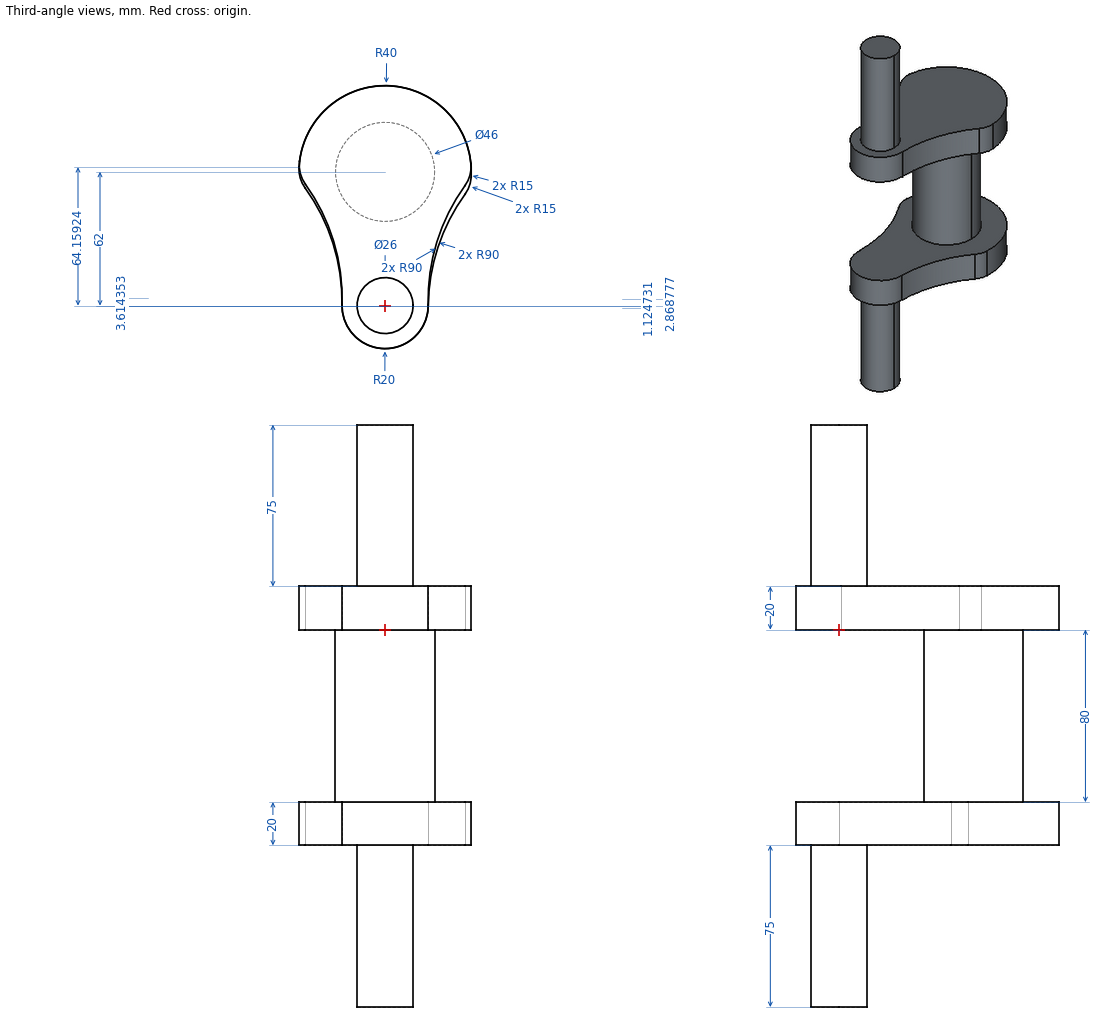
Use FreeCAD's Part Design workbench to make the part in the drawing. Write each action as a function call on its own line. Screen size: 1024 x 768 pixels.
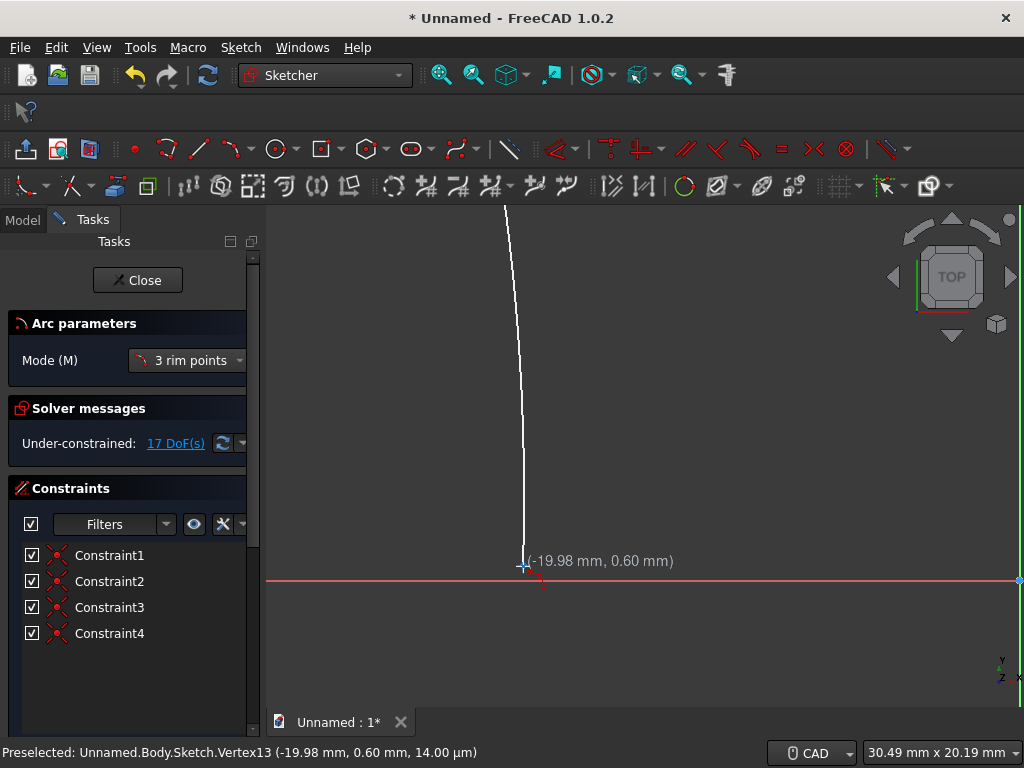
scroll(521, 567, down, 11)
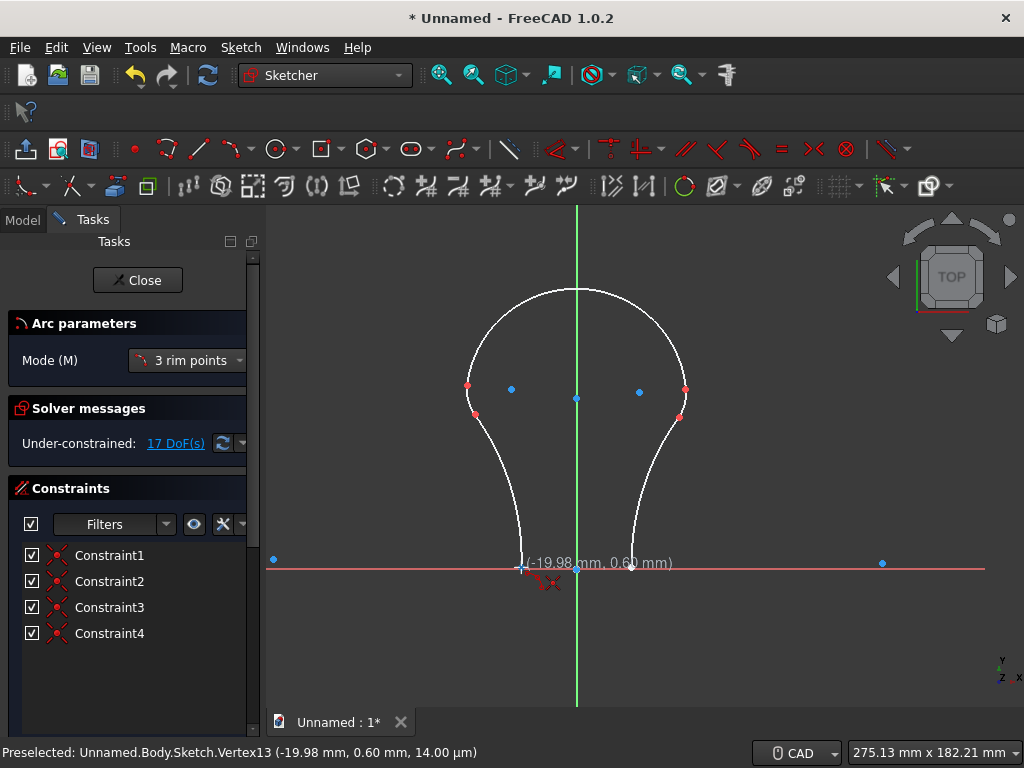
scroll(632, 568, up, 13)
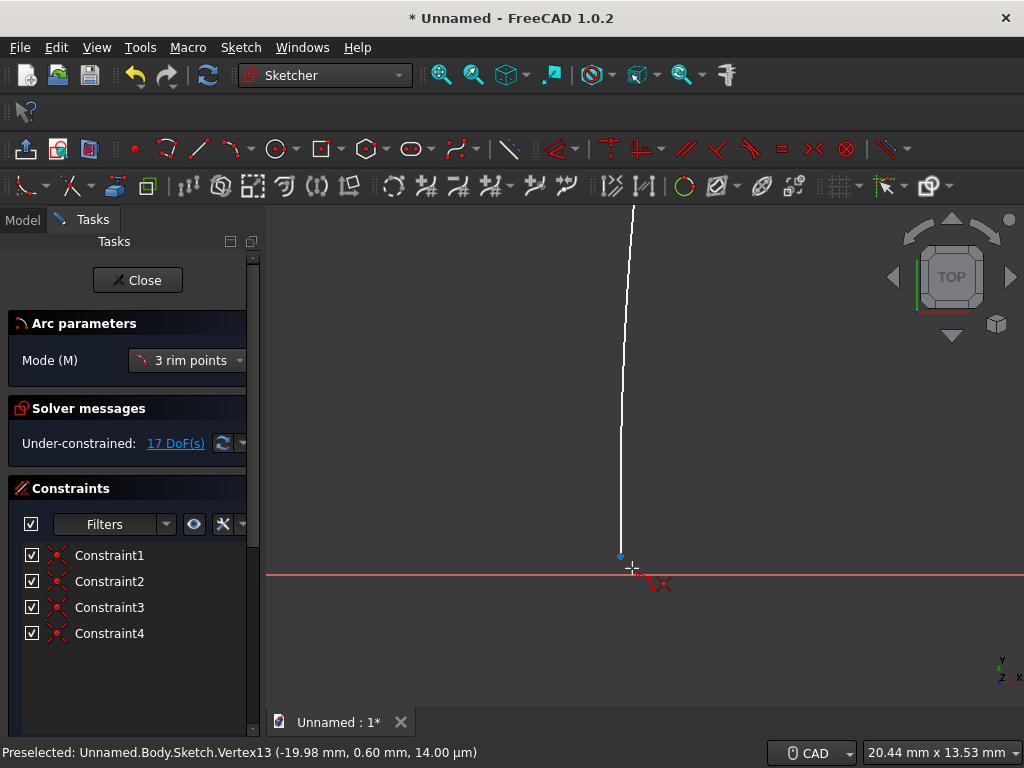
click(621, 557)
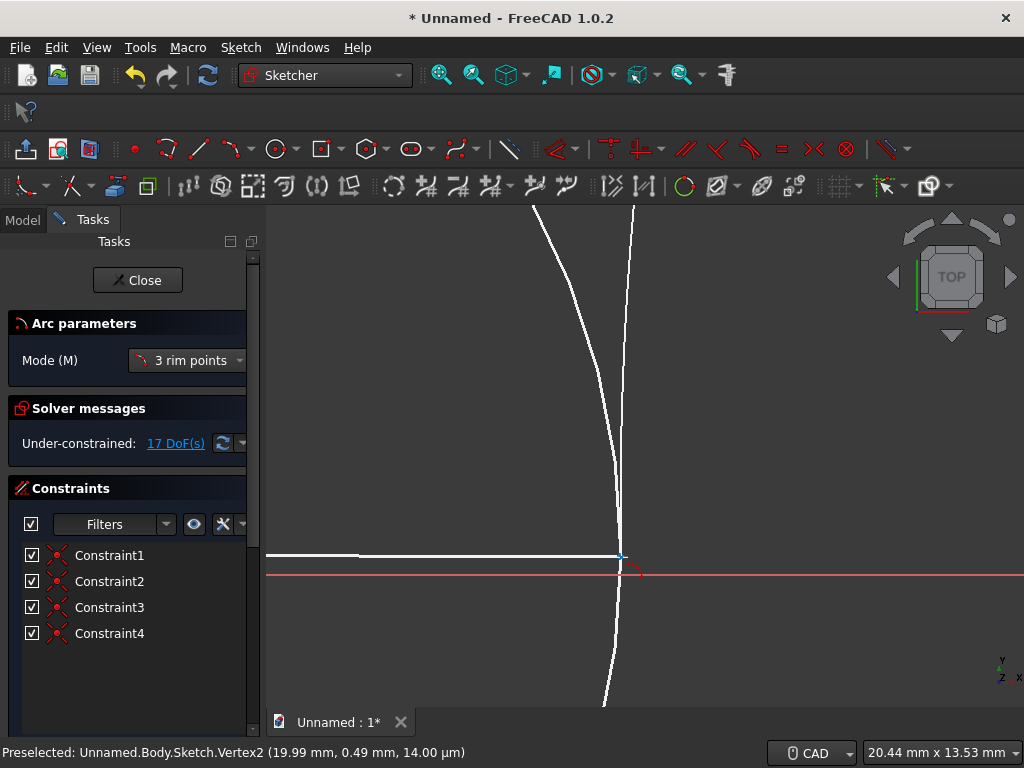
scroll(632, 568, down, 13)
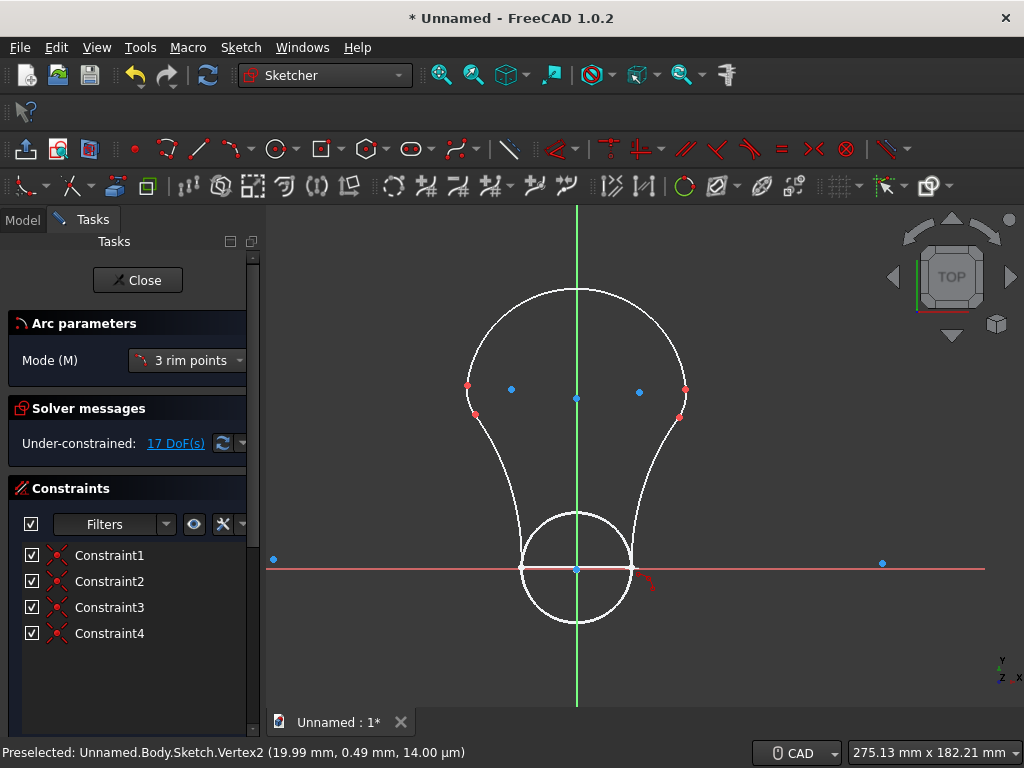
click(559, 621)
key(Escape)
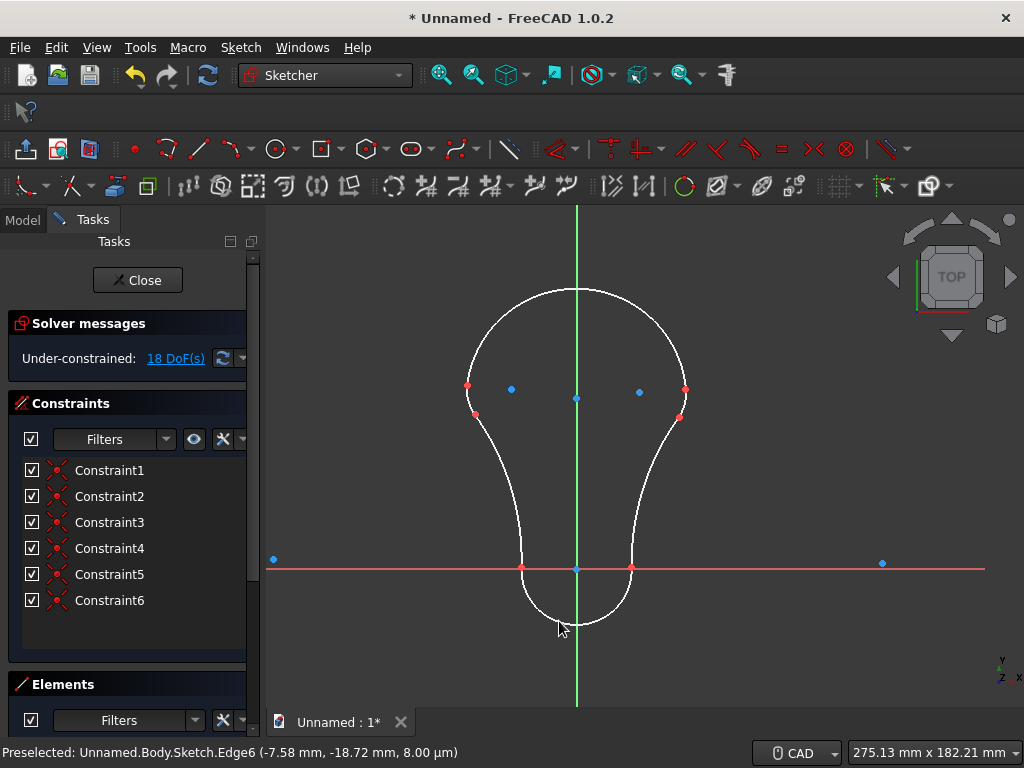
click(655, 459)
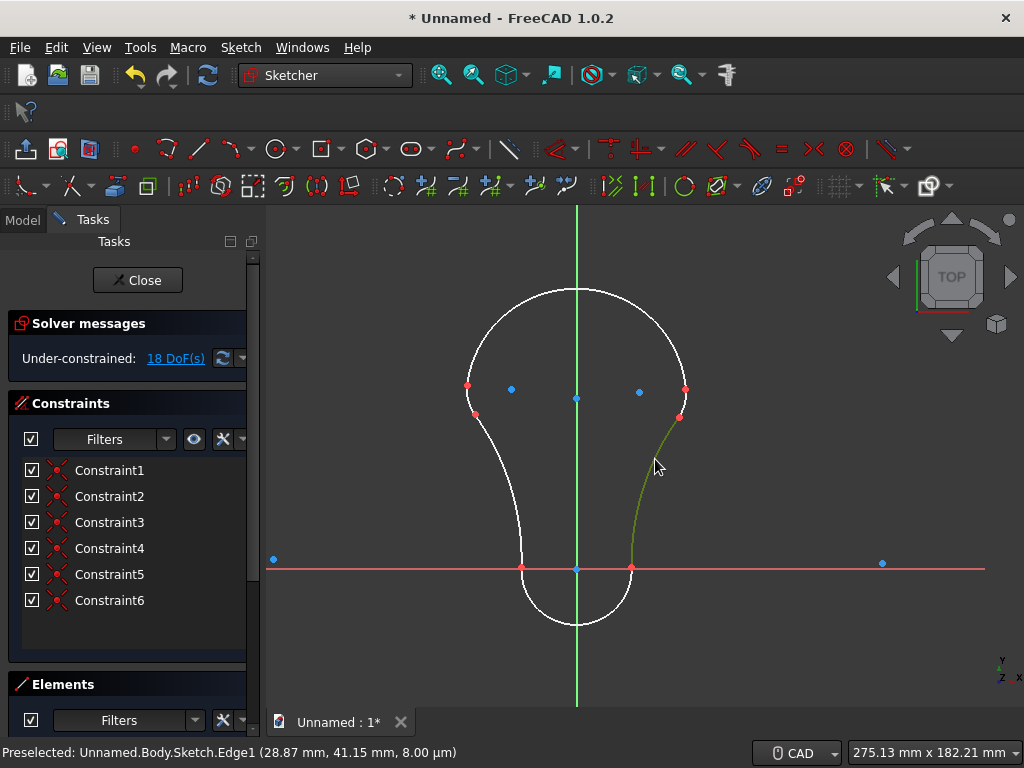
click(685, 404)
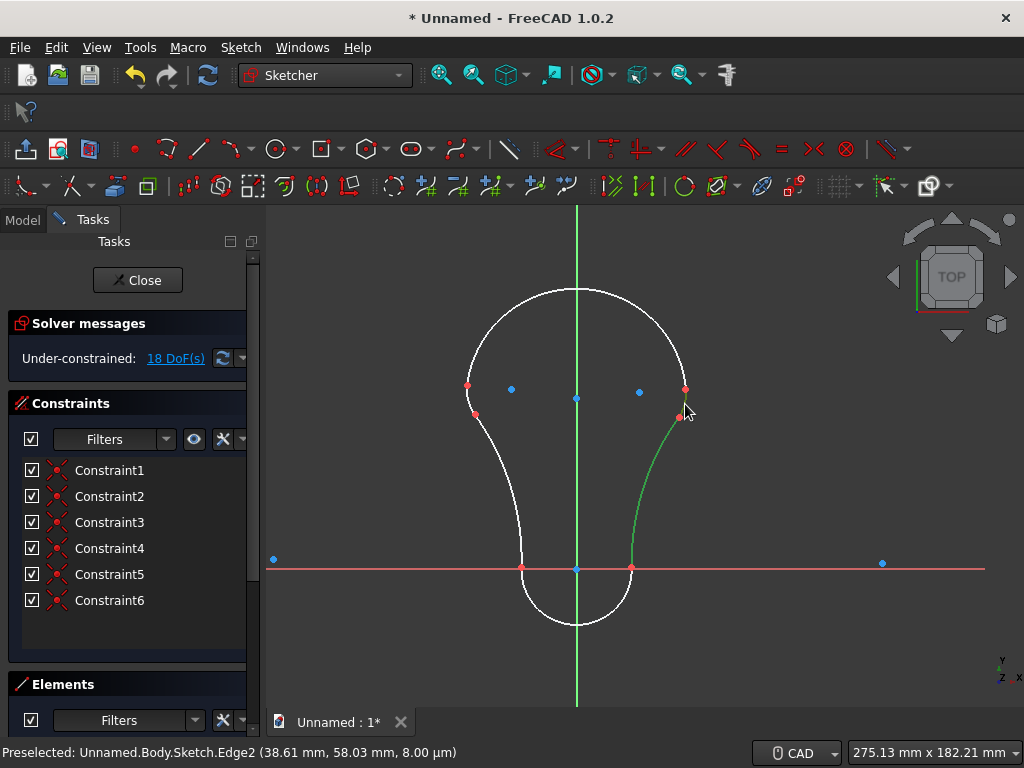
click(750, 150)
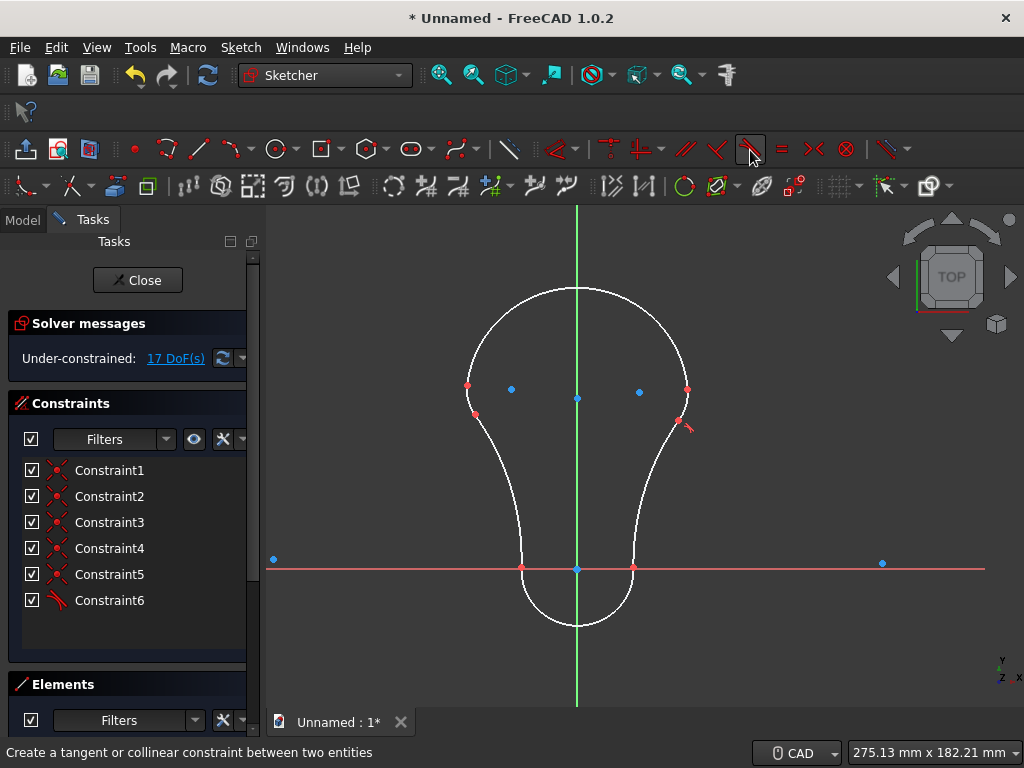
click(656, 461)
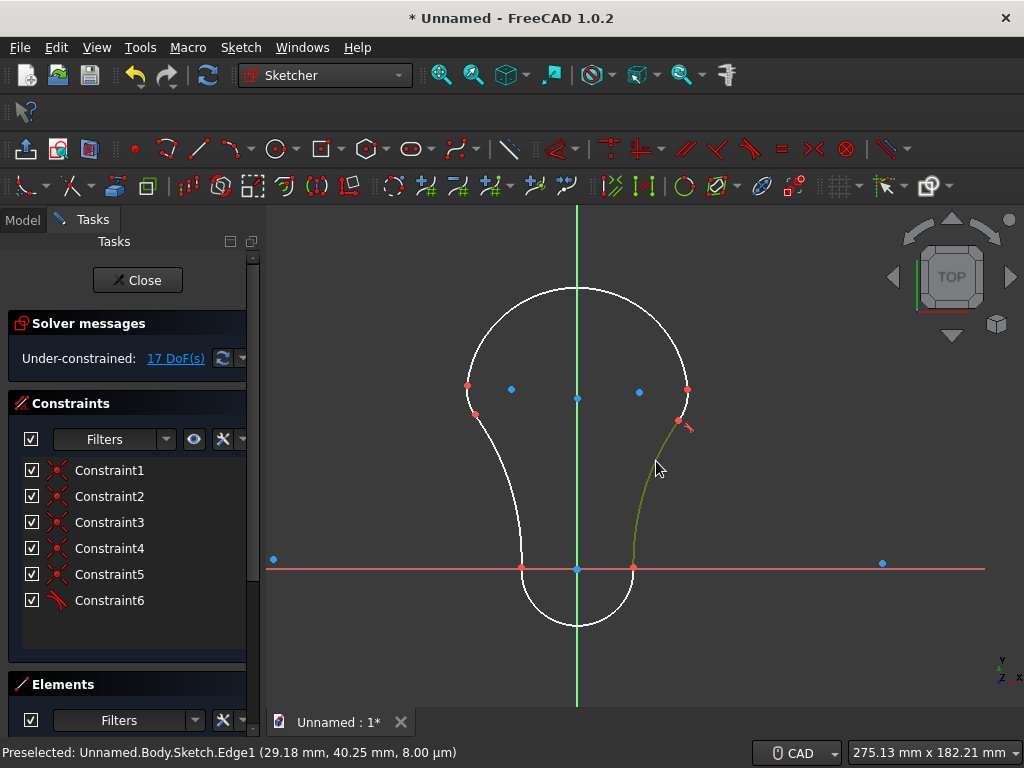
click(544, 615)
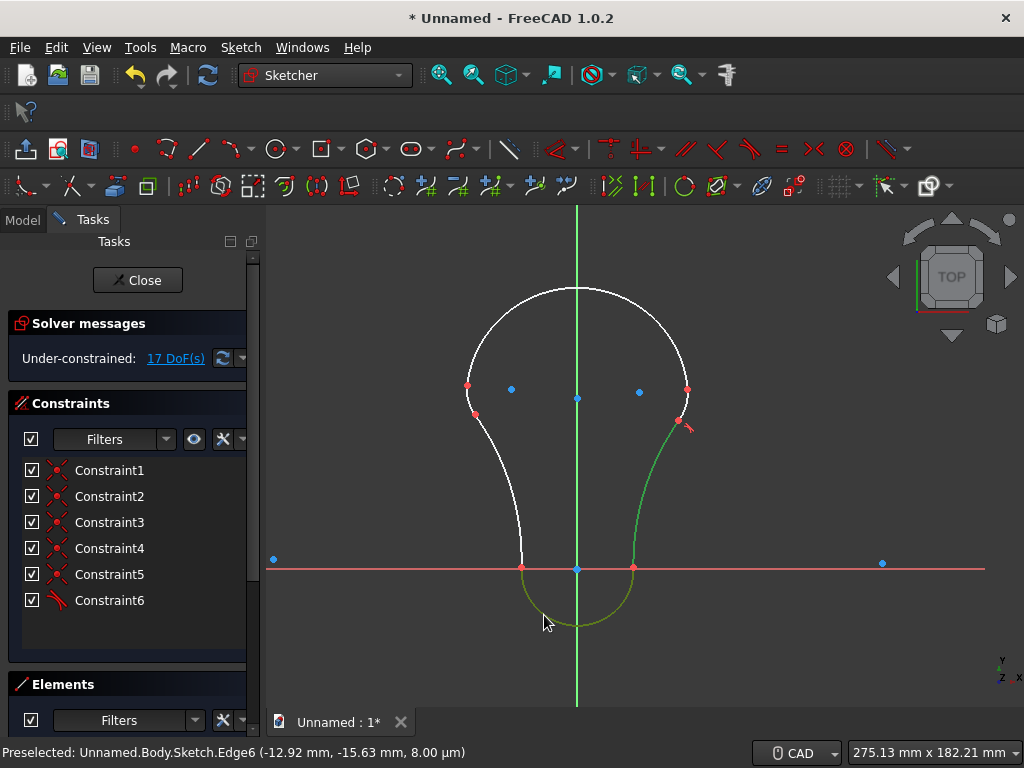
click(750, 150)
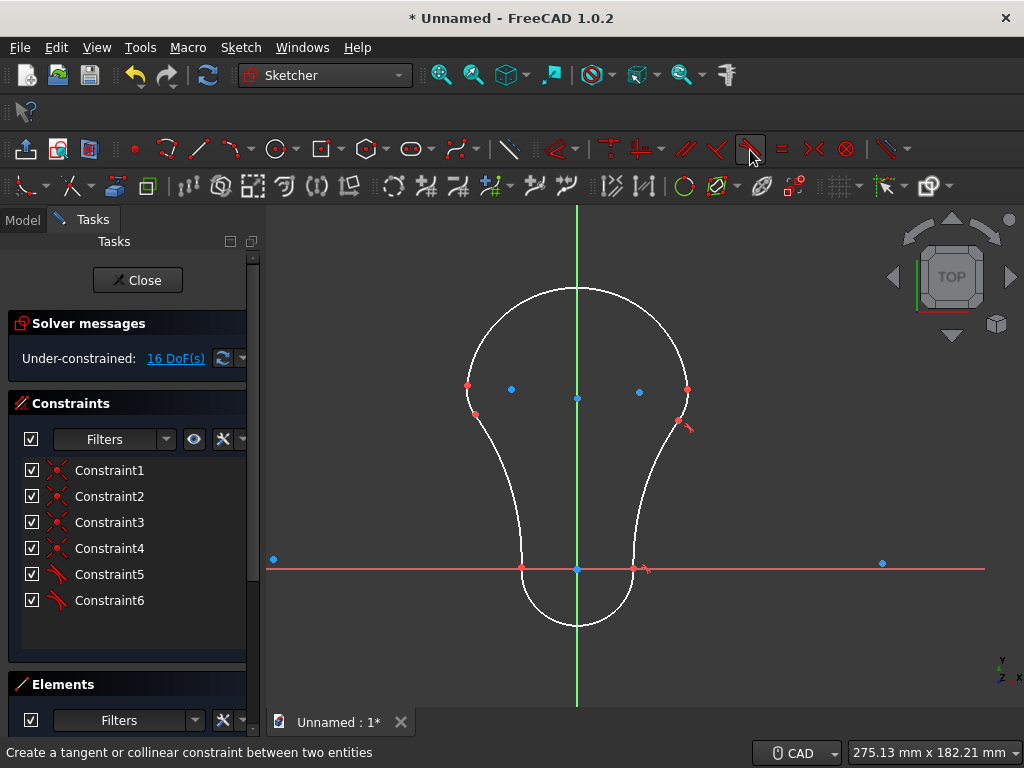
scroll(684, 412, up, 2)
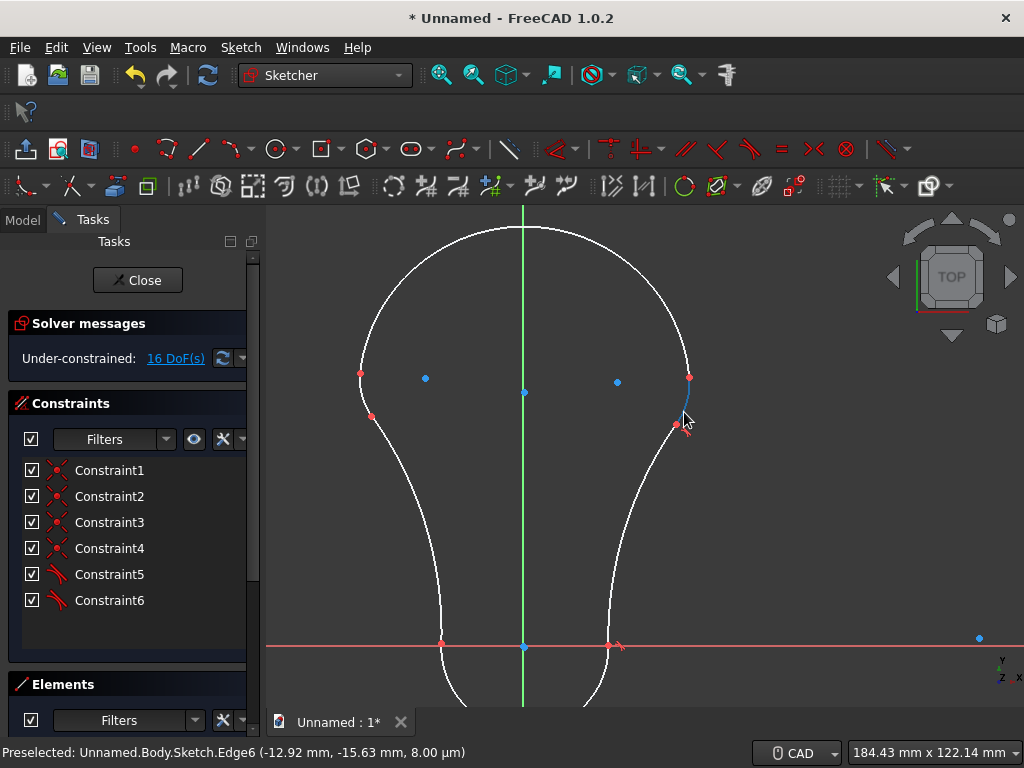
click(683, 411)